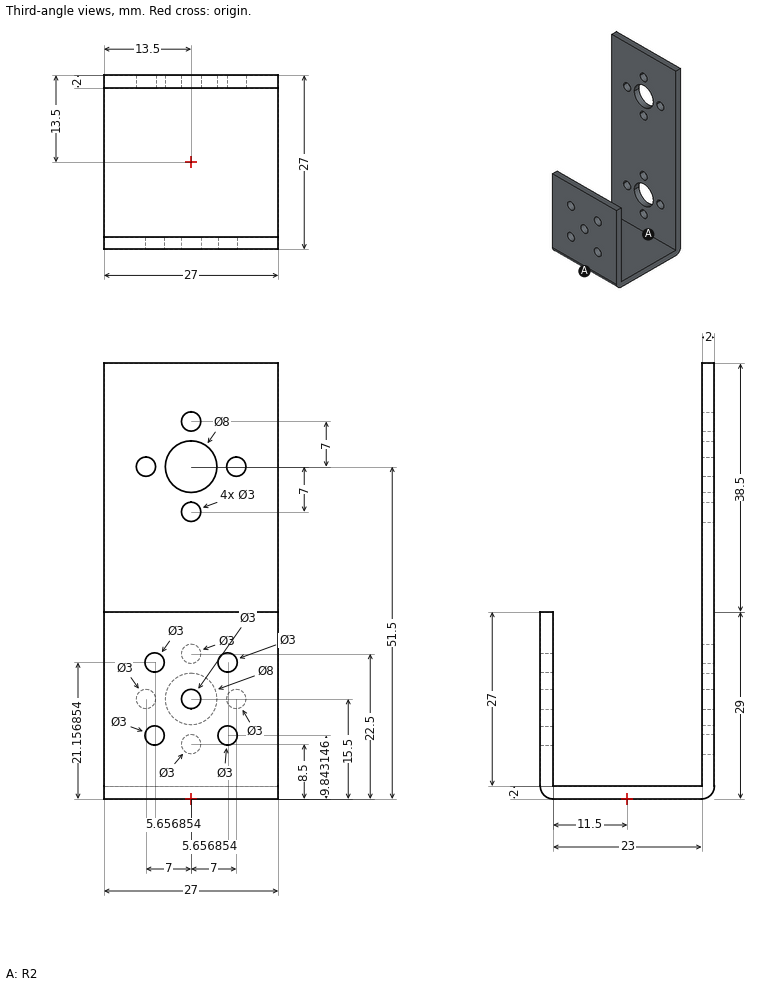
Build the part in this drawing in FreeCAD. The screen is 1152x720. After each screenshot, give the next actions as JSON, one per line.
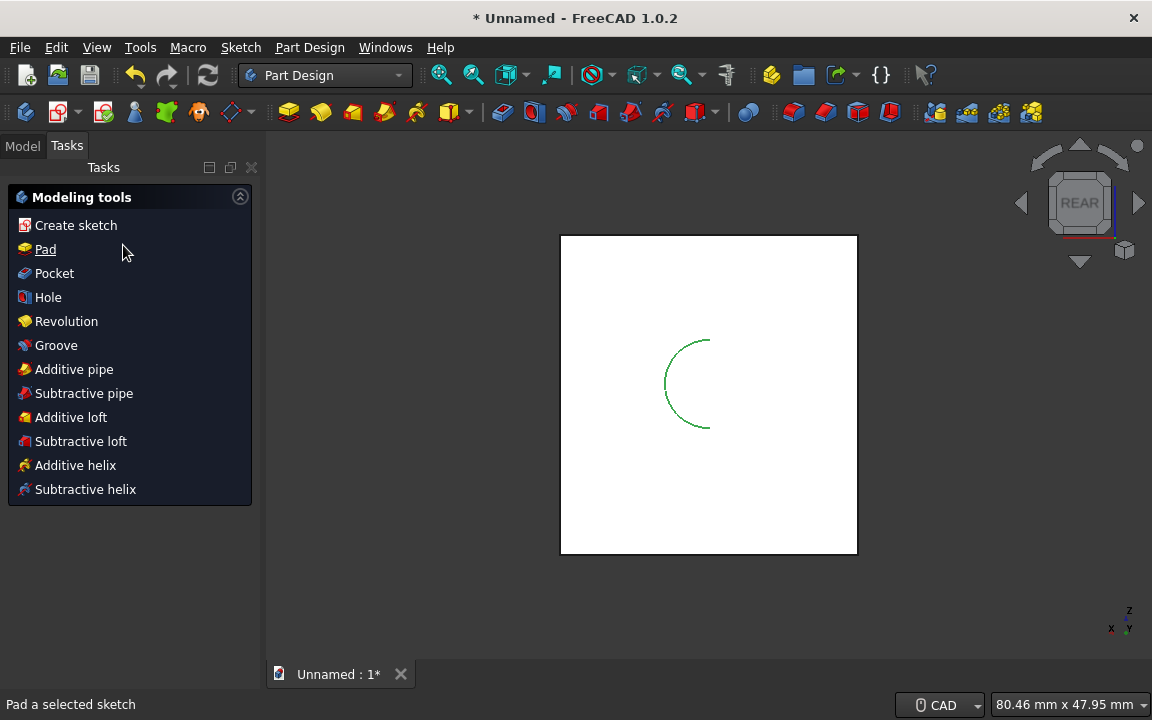
{"action": "left_click", "coordinate": [504, 112]}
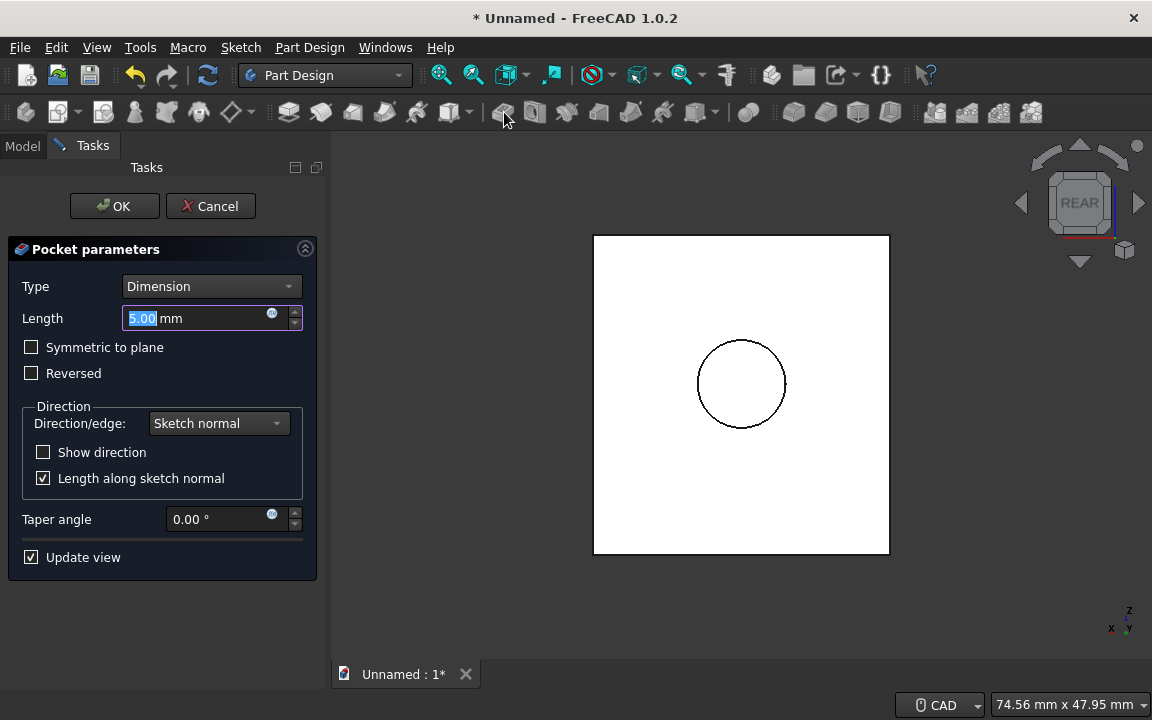
{"action": "left_click", "coordinate": [212, 286]}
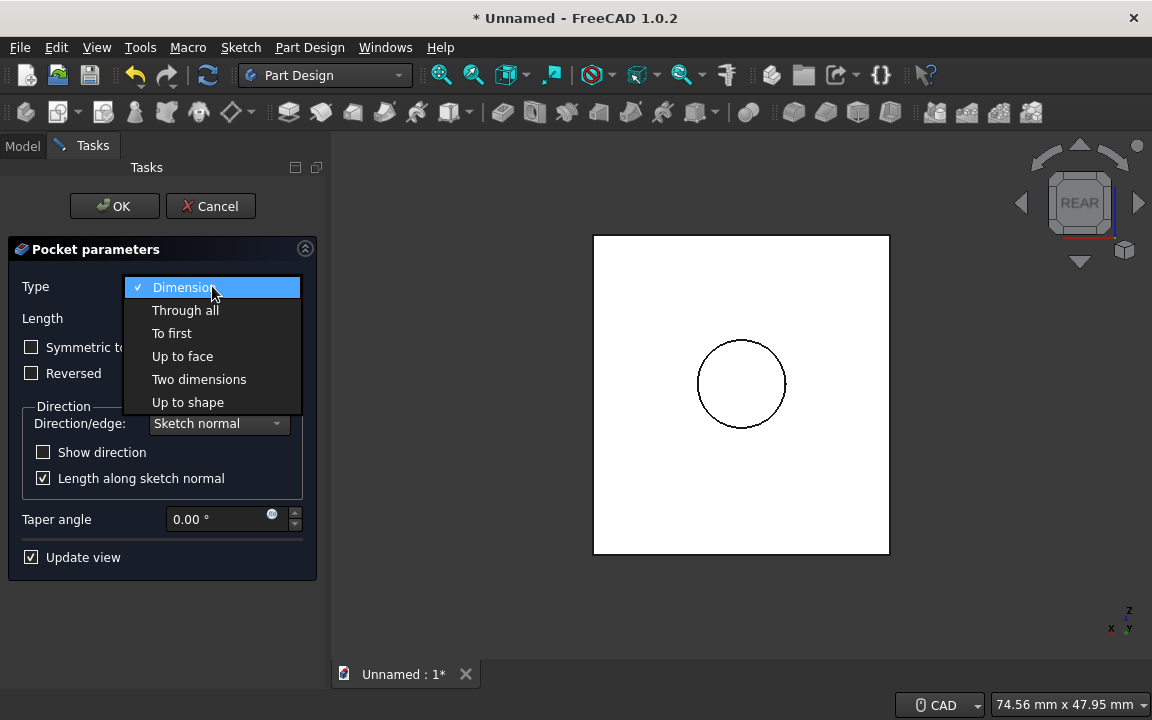
{"action": "left_click", "coordinate": [212, 334]}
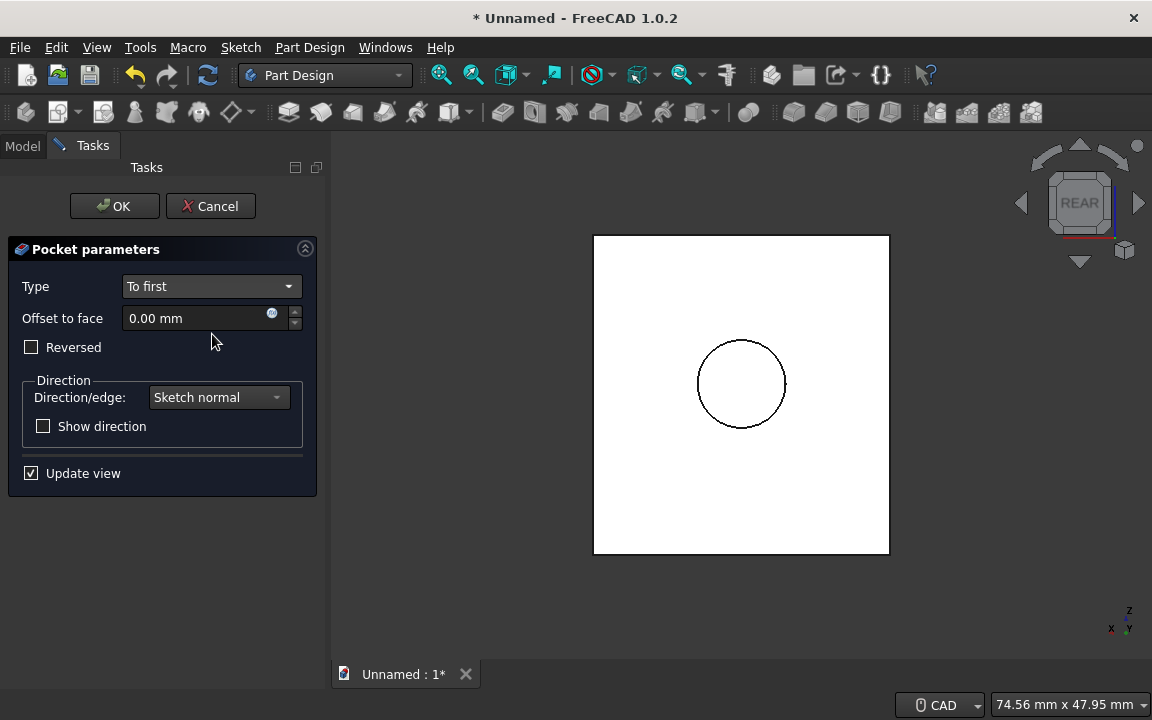
{"action": "left_click", "coordinate": [115, 206]}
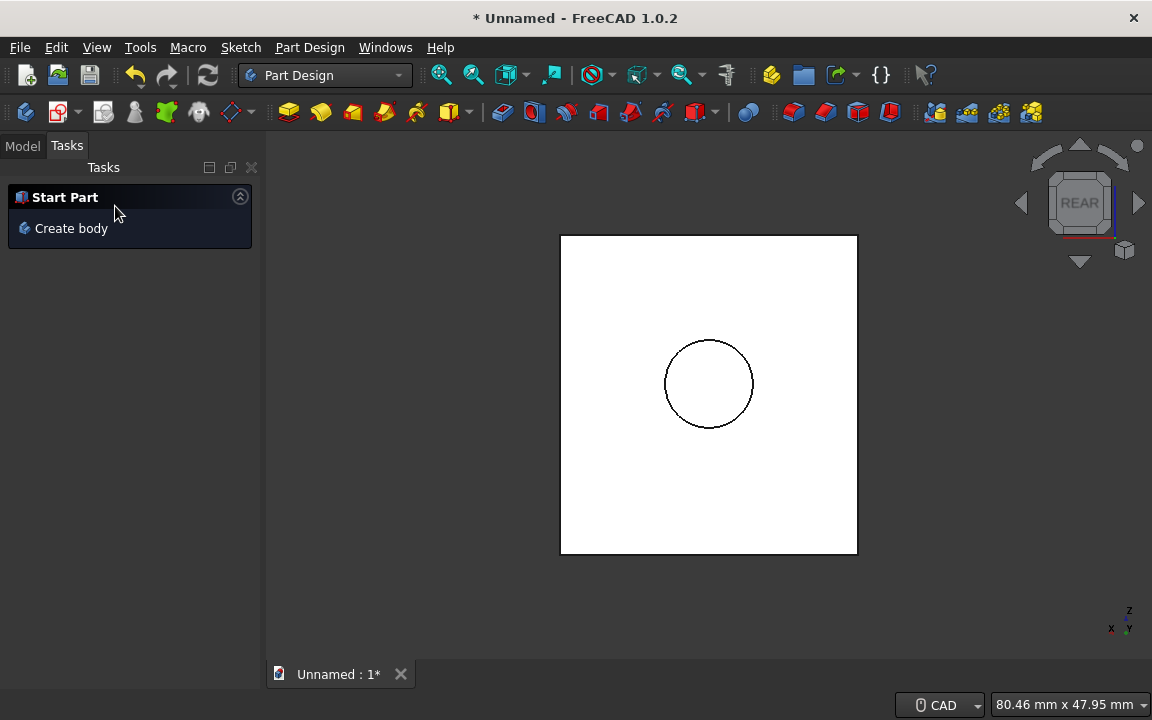
{"action": "left_click", "coordinate": [751, 485]}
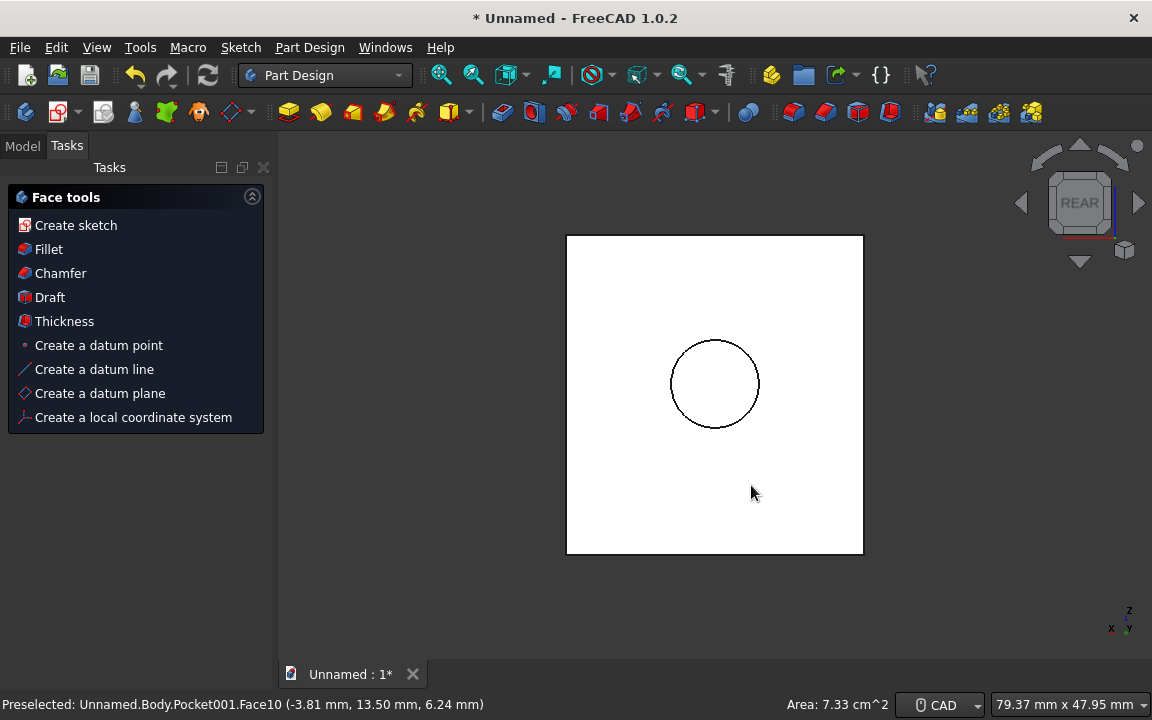
{"action": "left_click", "coordinate": [58, 112]}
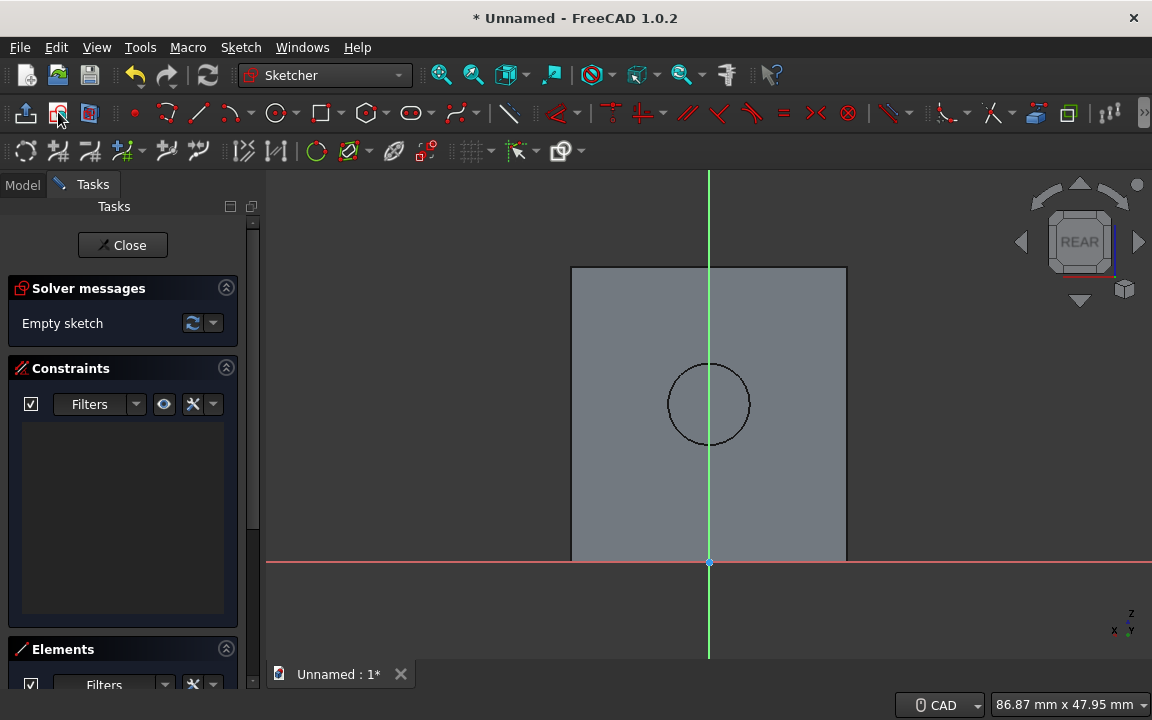
{"action": "scroll", "coordinate": [716, 482], "scroll_direction": "up", "scroll_amount": 12}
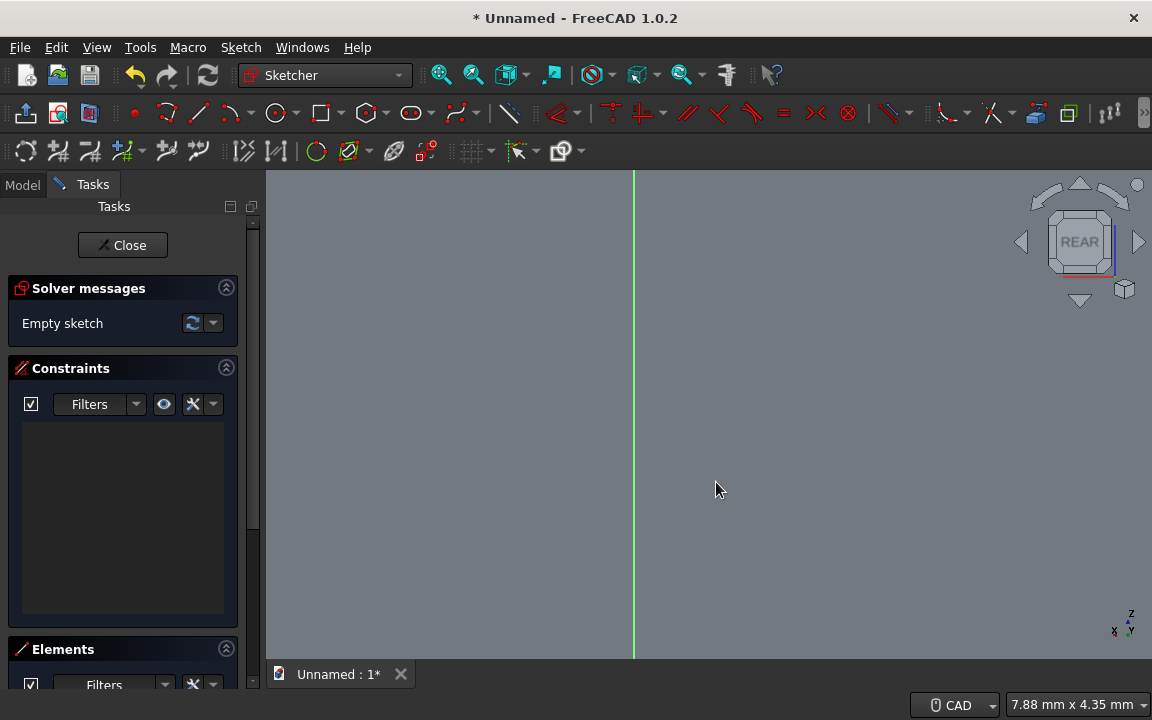
{"action": "left_click", "coordinate": [276, 114]}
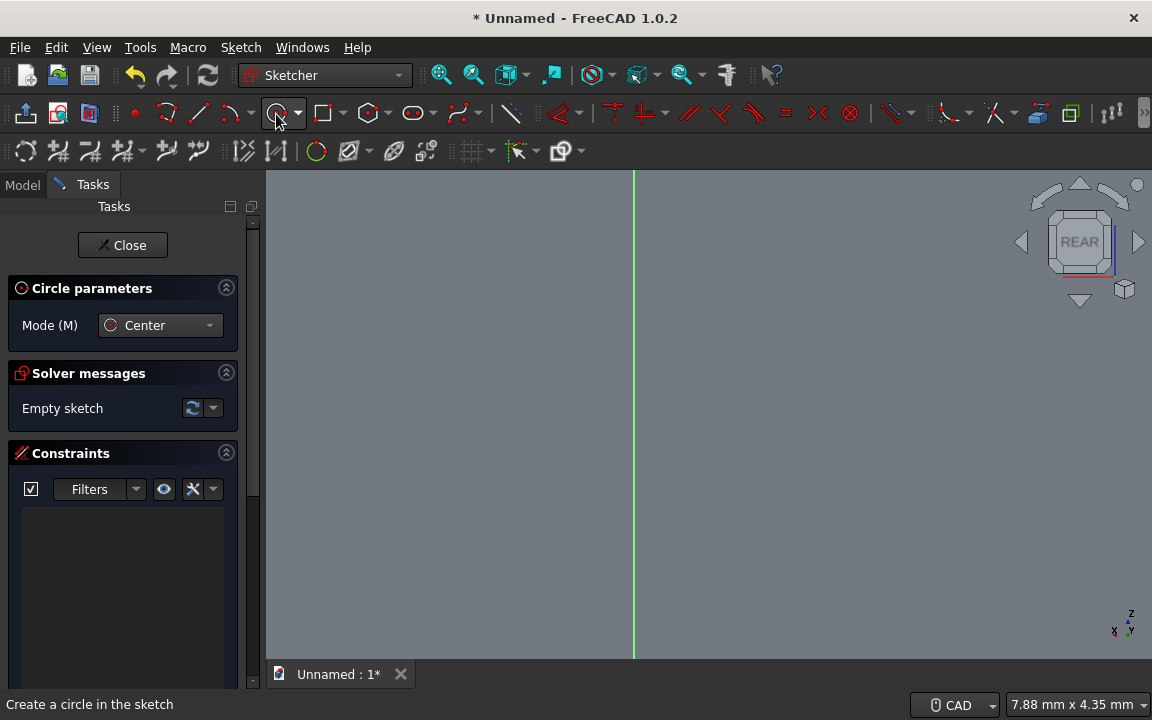
{"action": "left_click", "coordinate": [634, 406]}
{"action": "left_click", "coordinate": [753, 287]}
{"action": "key", "text": "Escape"}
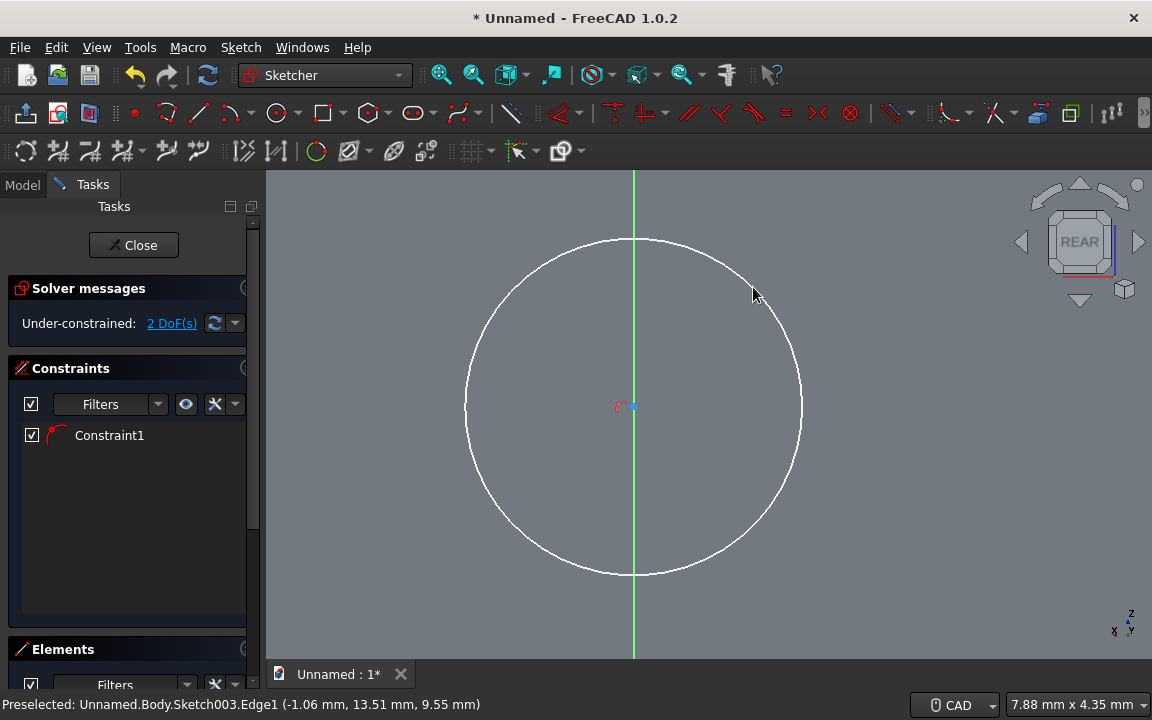
{"action": "key", "text": "d"}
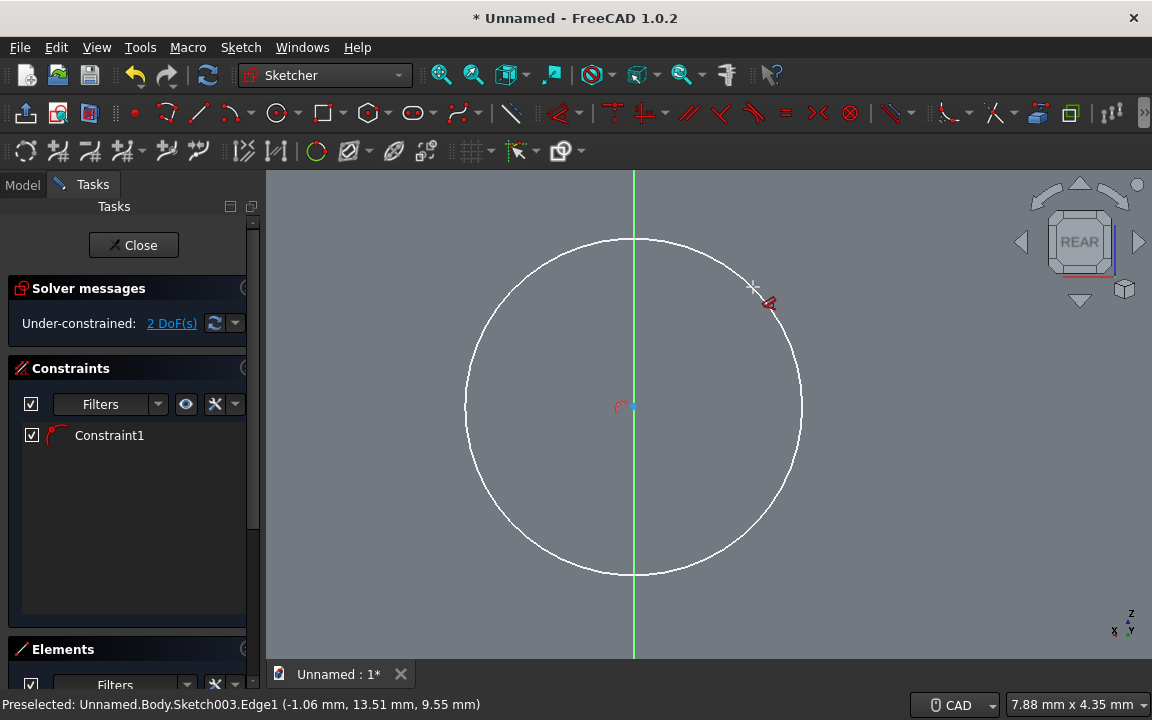
{"action": "left_click", "coordinate": [753, 288]}
{"action": "left_click", "coordinate": [776, 265]}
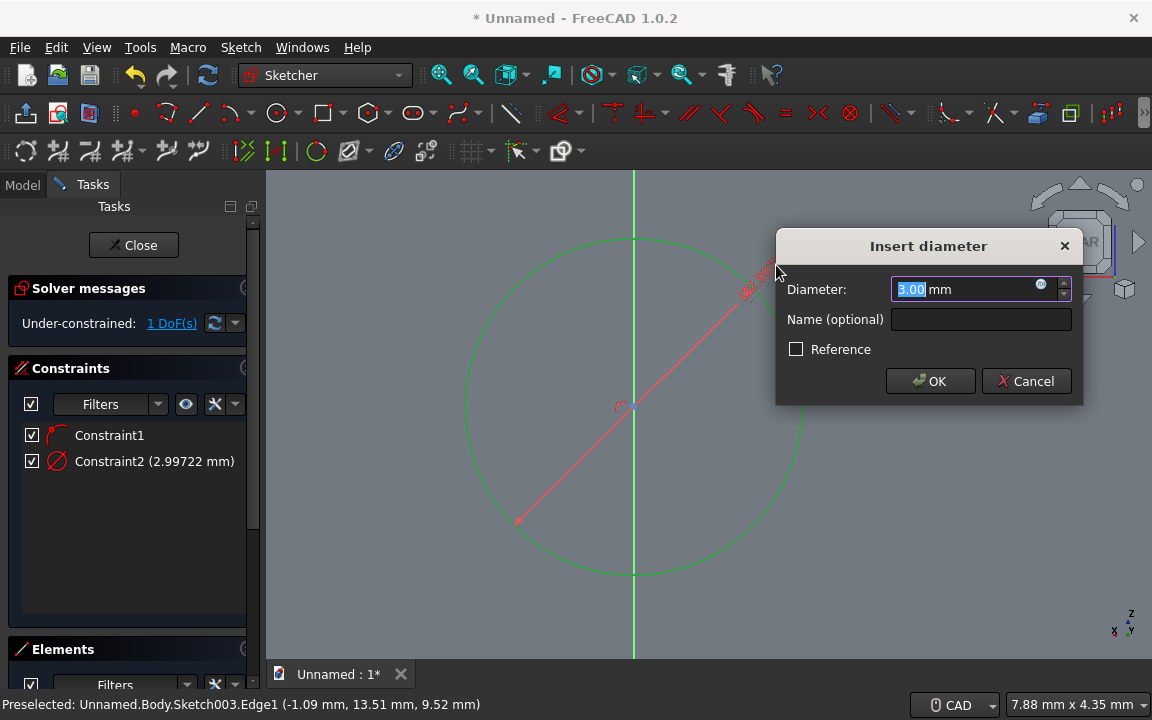
{"action": "type", "text": "3"}
{"action": "key", "text": "Return"}